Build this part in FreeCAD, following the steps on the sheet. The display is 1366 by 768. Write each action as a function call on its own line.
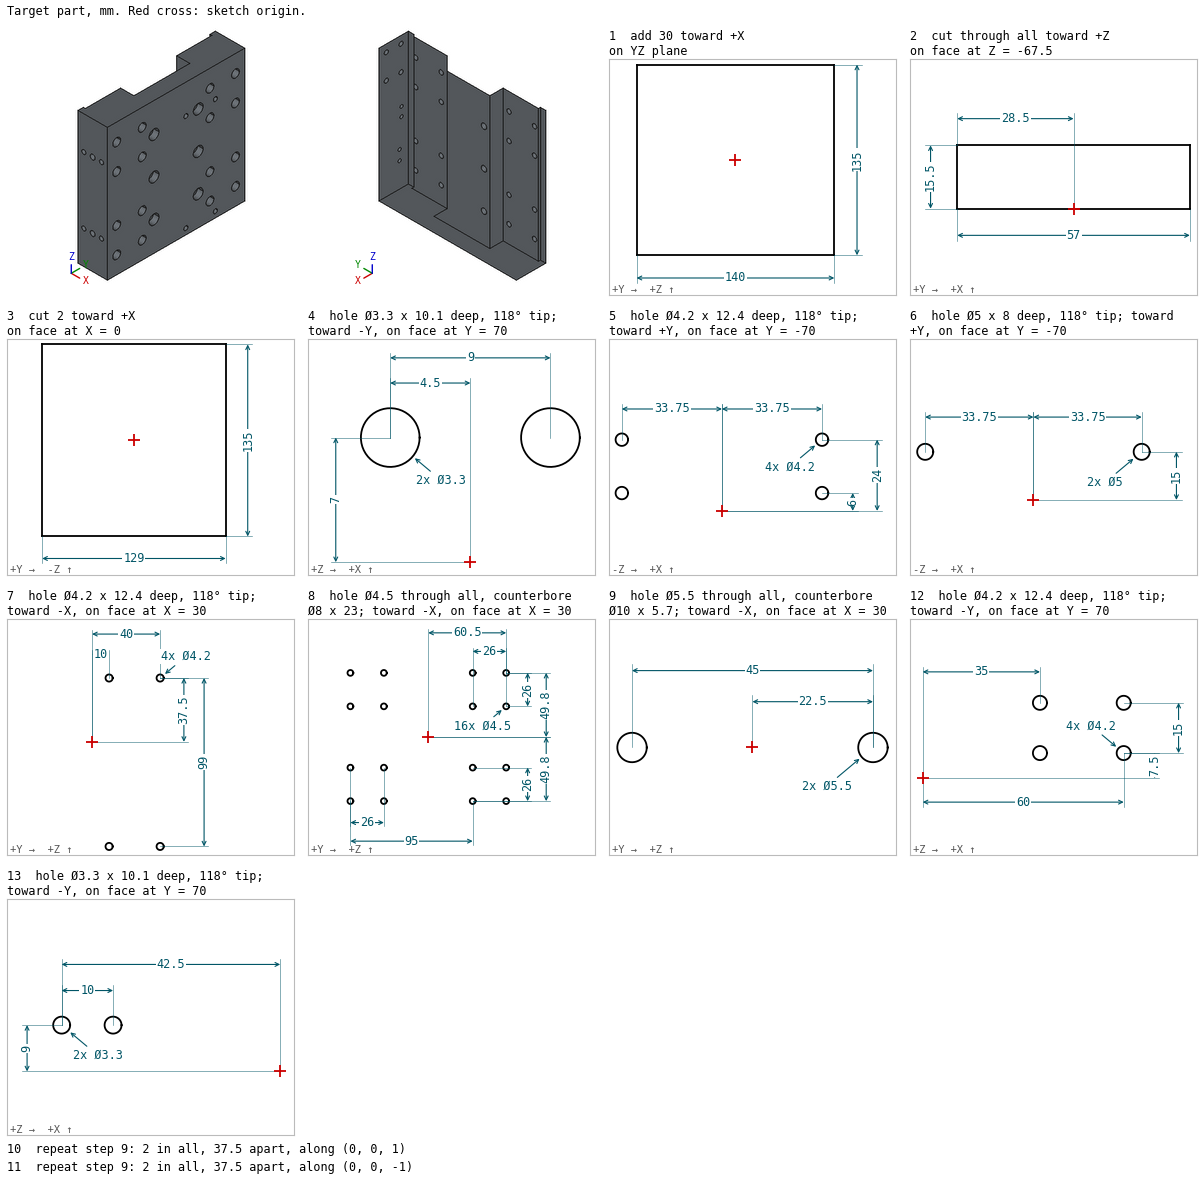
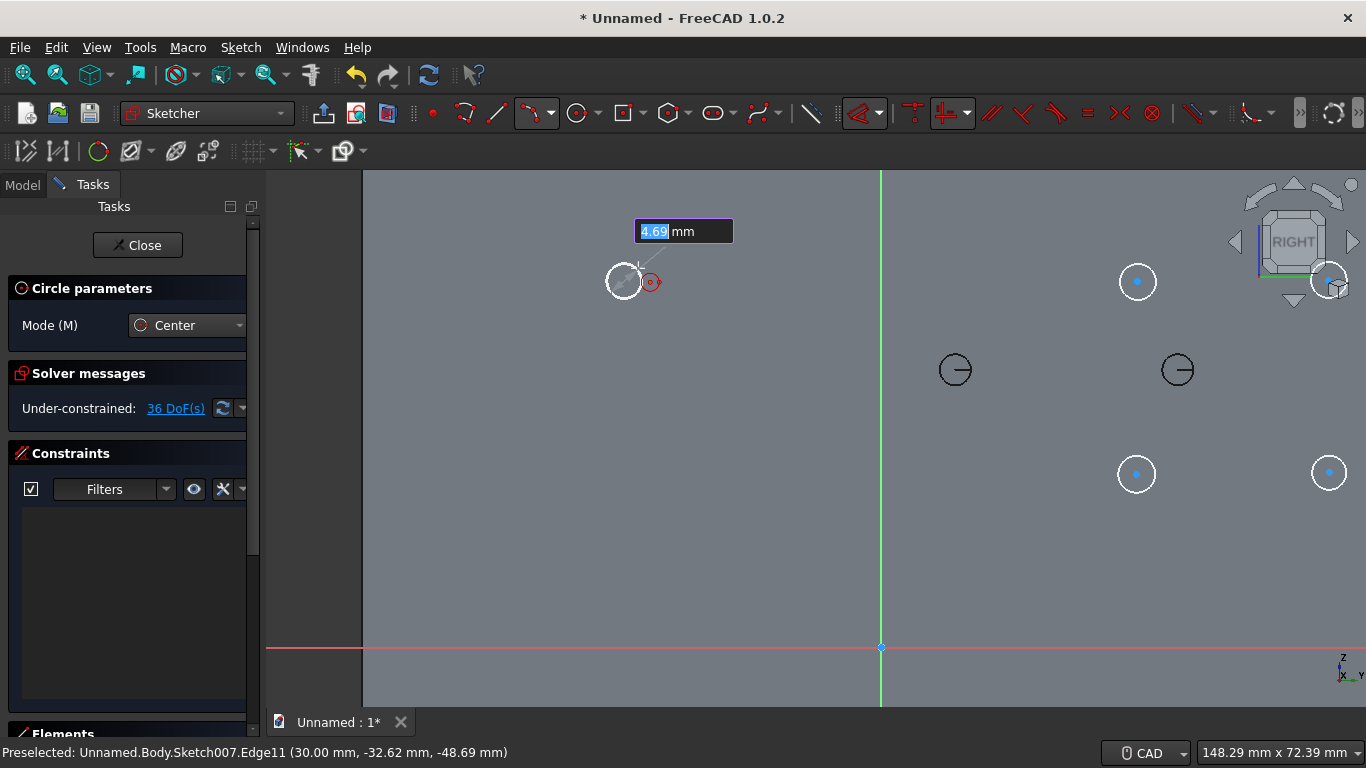
click(637, 267)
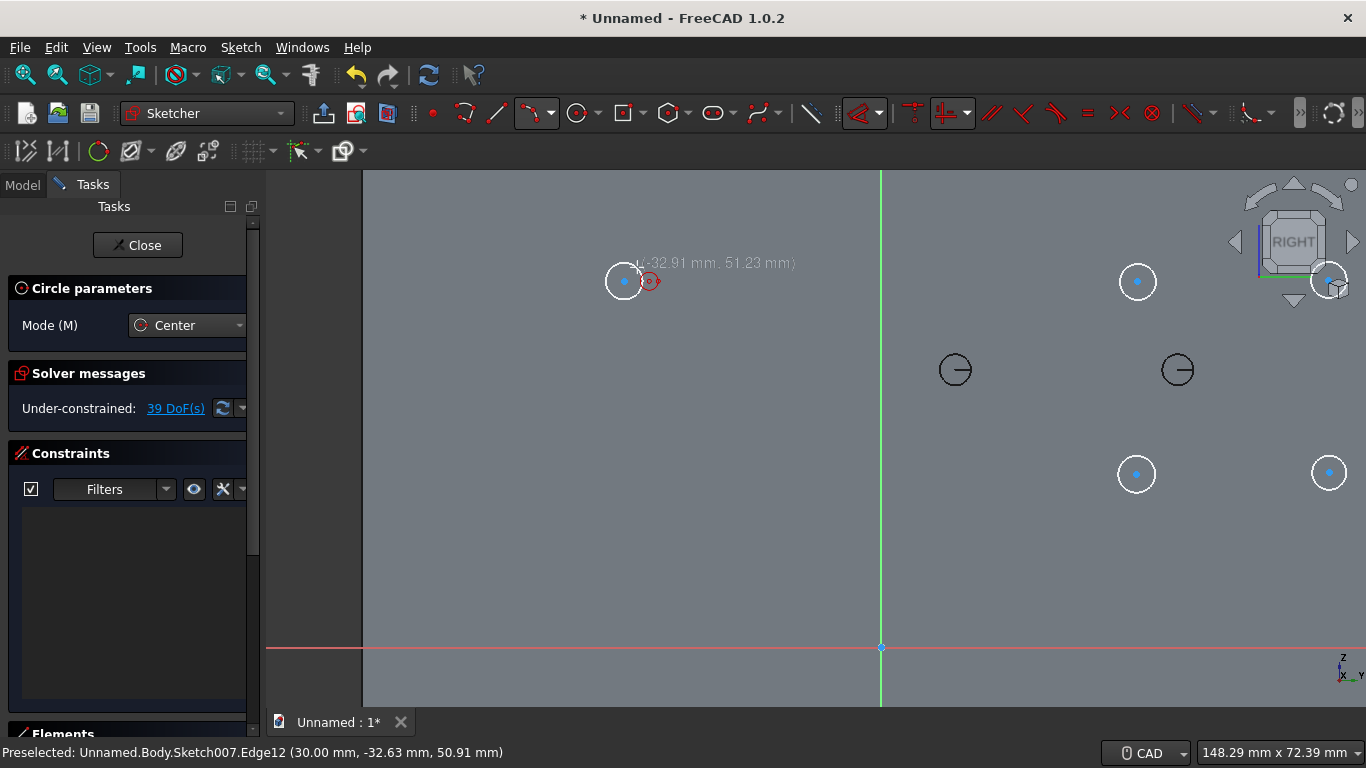
scroll(625, 471, up, 2)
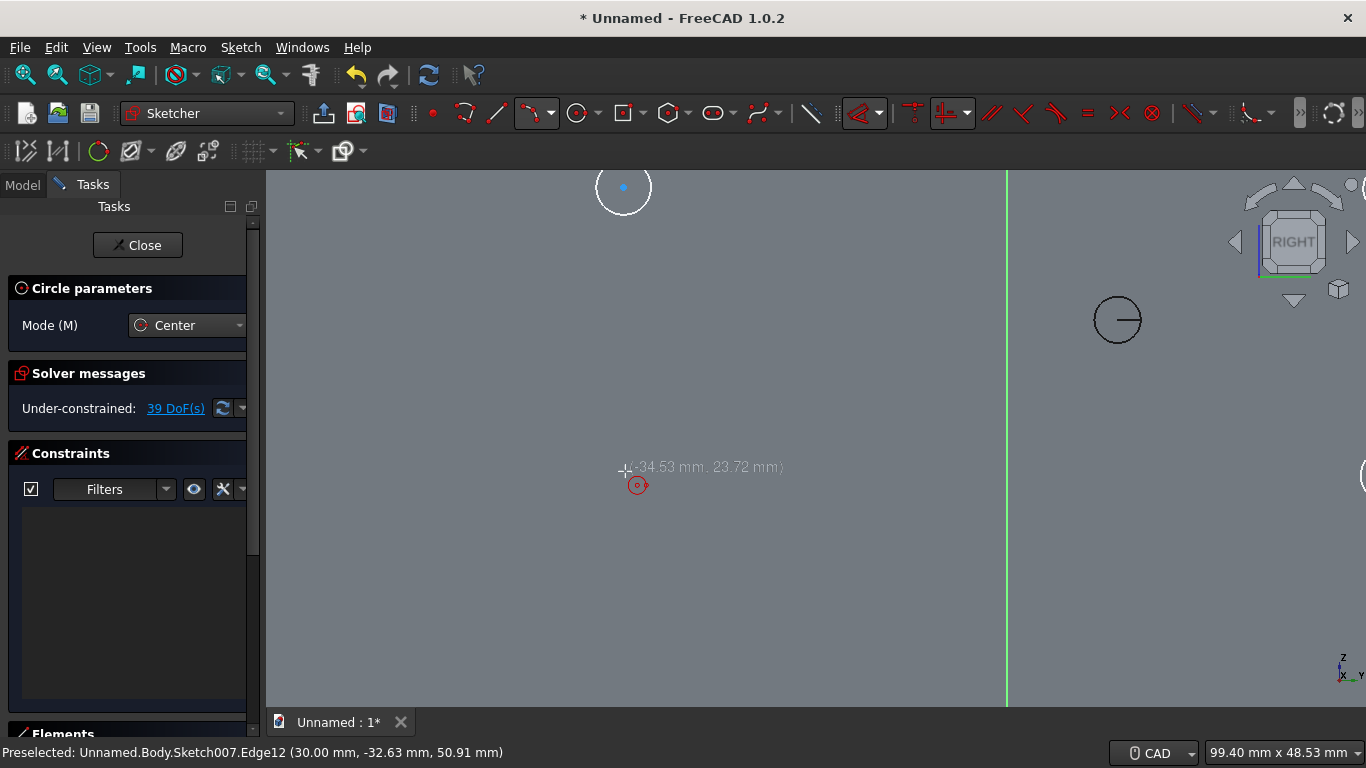
scroll(636, 311, down, 6)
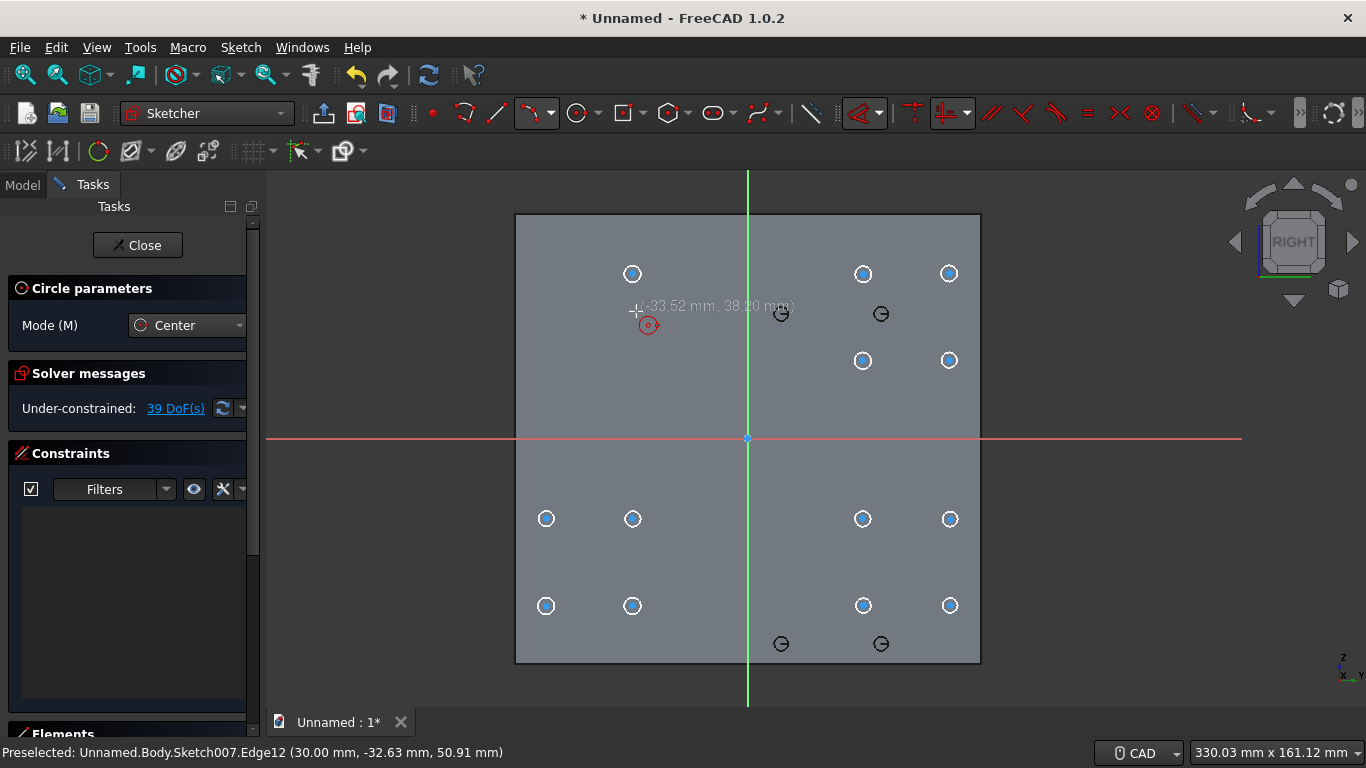
click(633, 359)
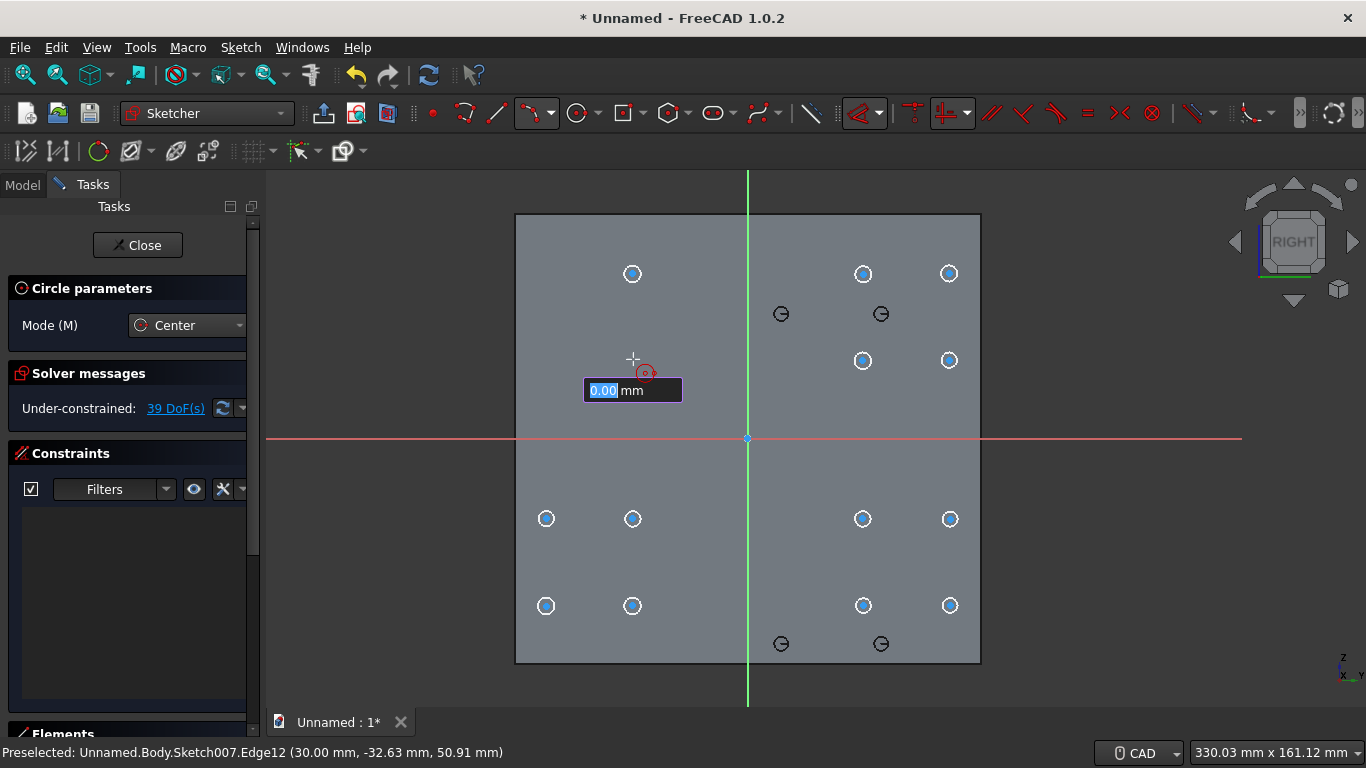
scroll(638, 354, up, 4)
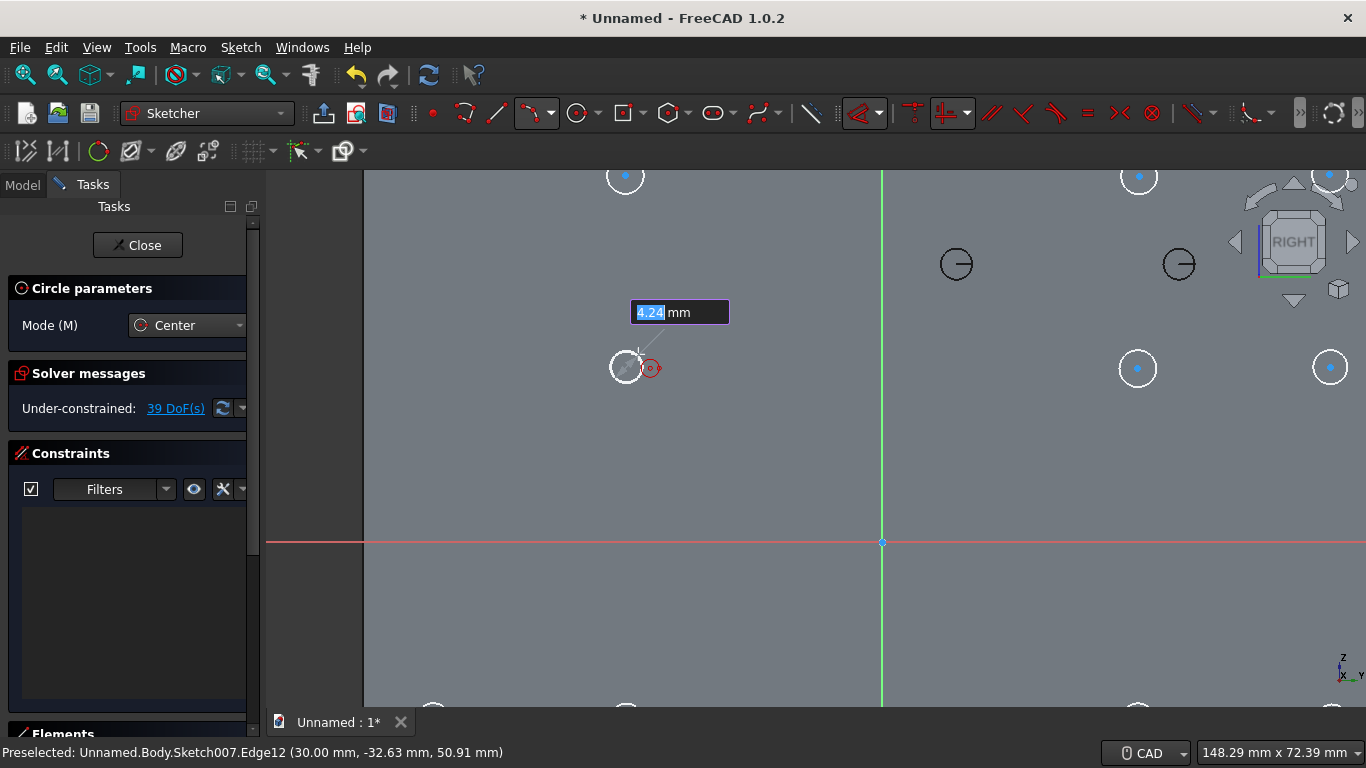
click(638, 354)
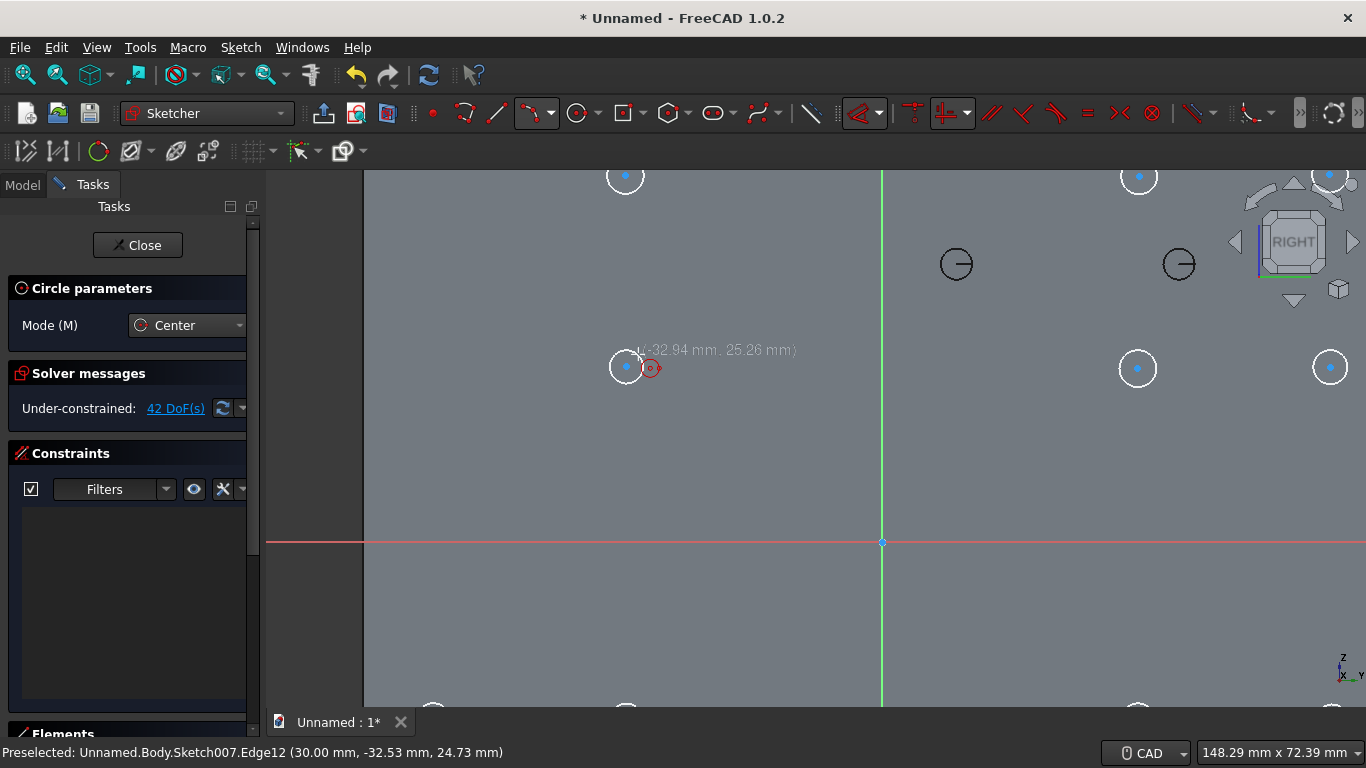
scroll(434, 366, up, 2)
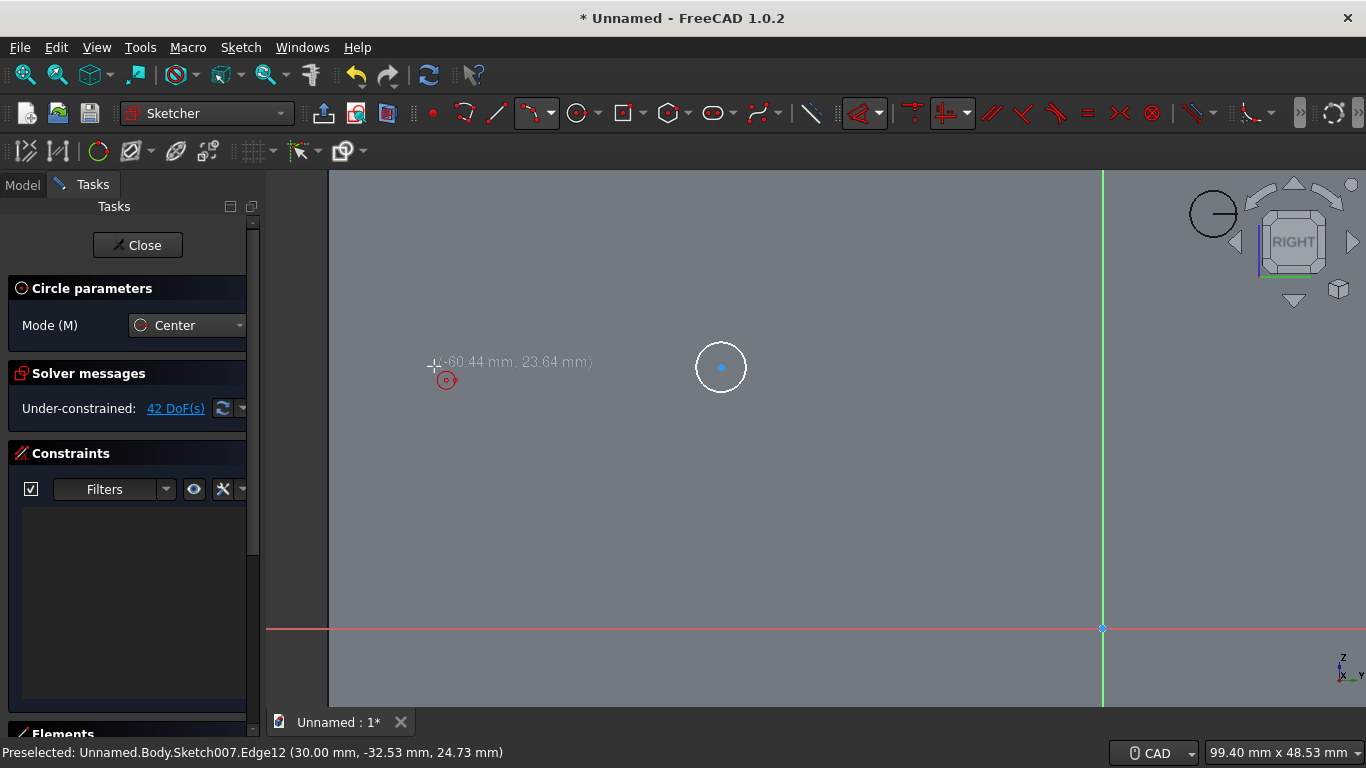
scroll(594, 356, down, 6)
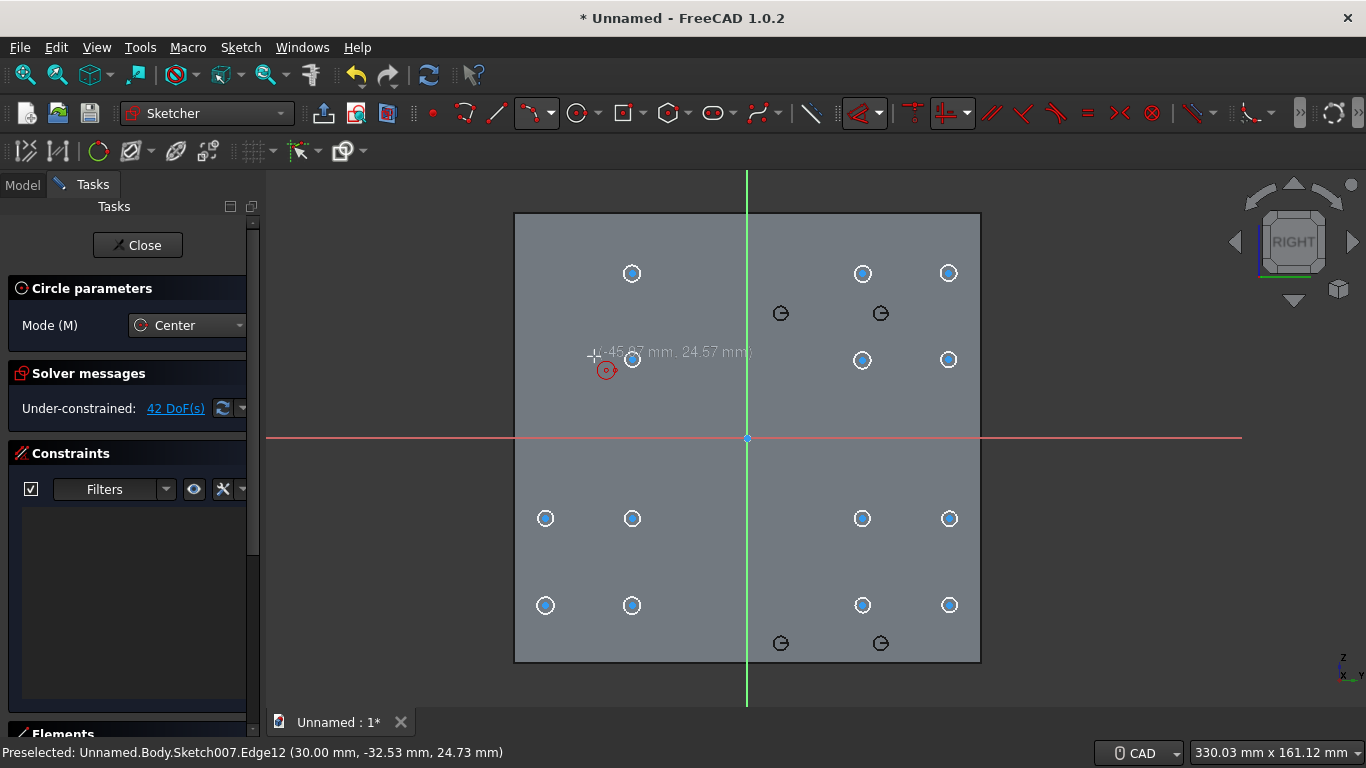
click(546, 359)